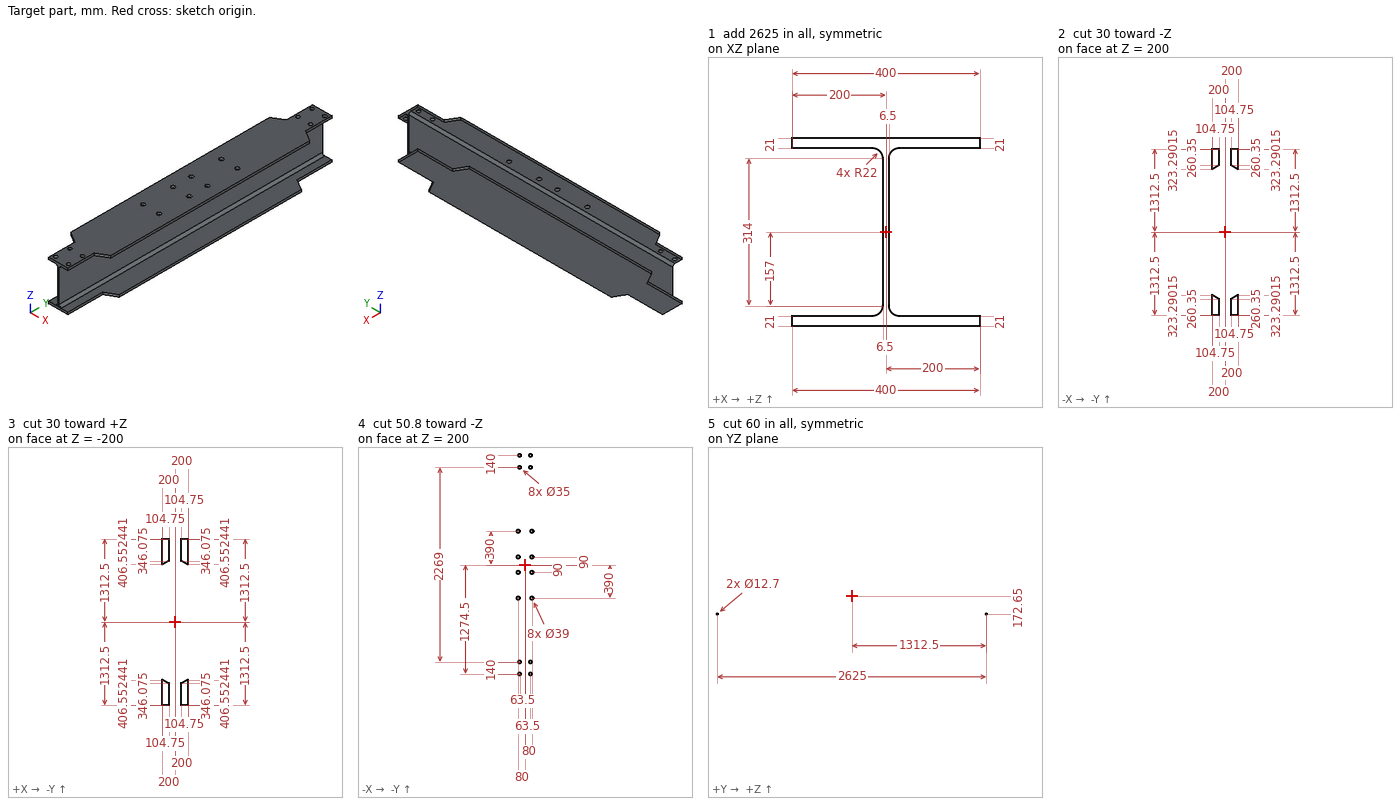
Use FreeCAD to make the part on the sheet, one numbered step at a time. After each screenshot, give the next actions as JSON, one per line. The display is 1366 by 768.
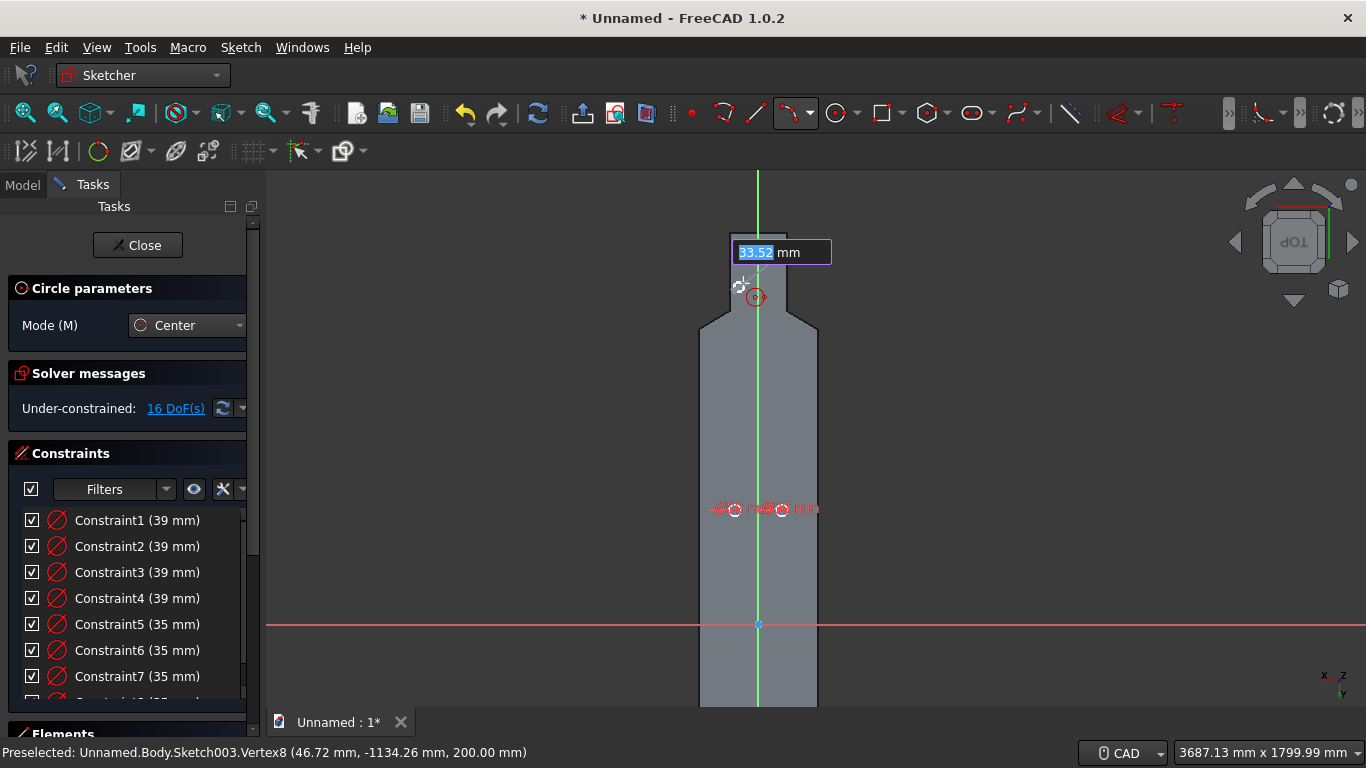
{"action": "type", "text": "35"}
{"action": "key", "text": "Return"}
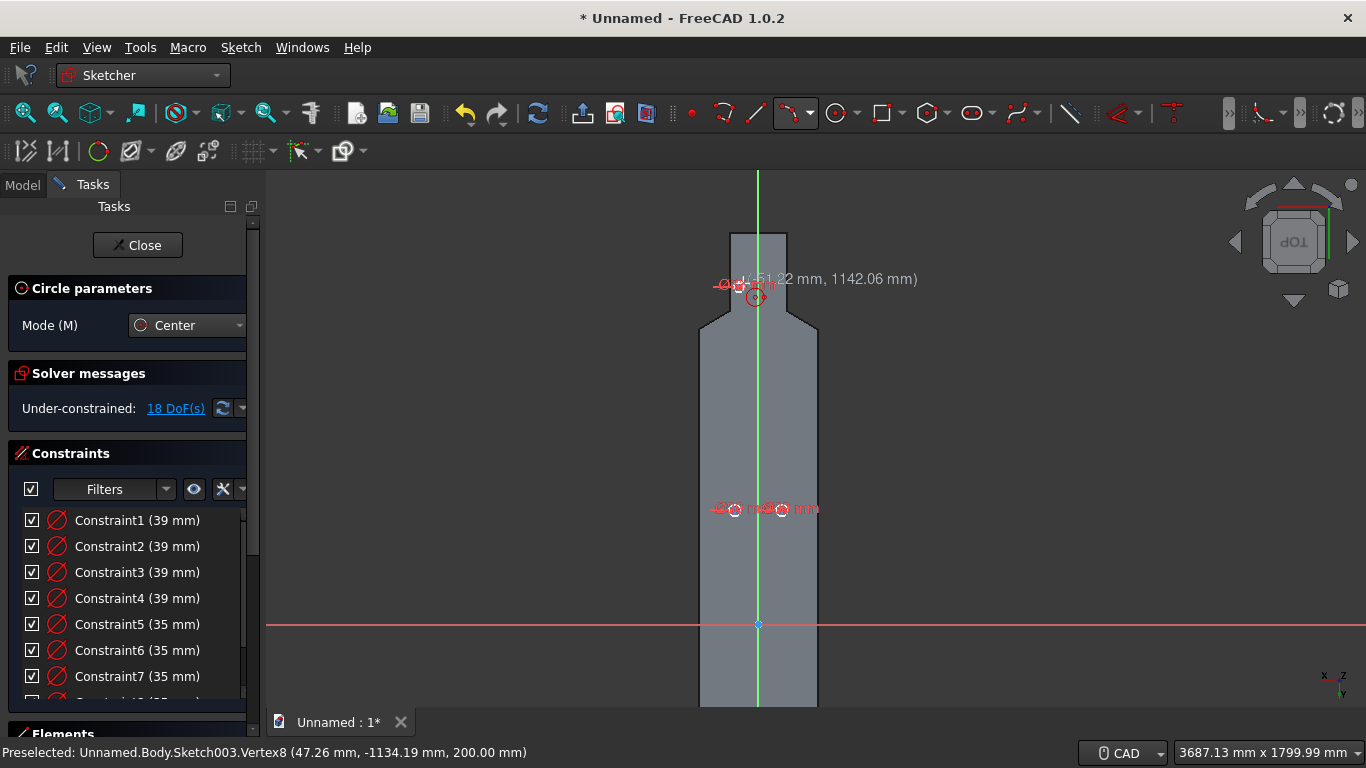
{"action": "scroll", "coordinate": [777, 286], "scroll_direction": "up", "scroll_amount": 8}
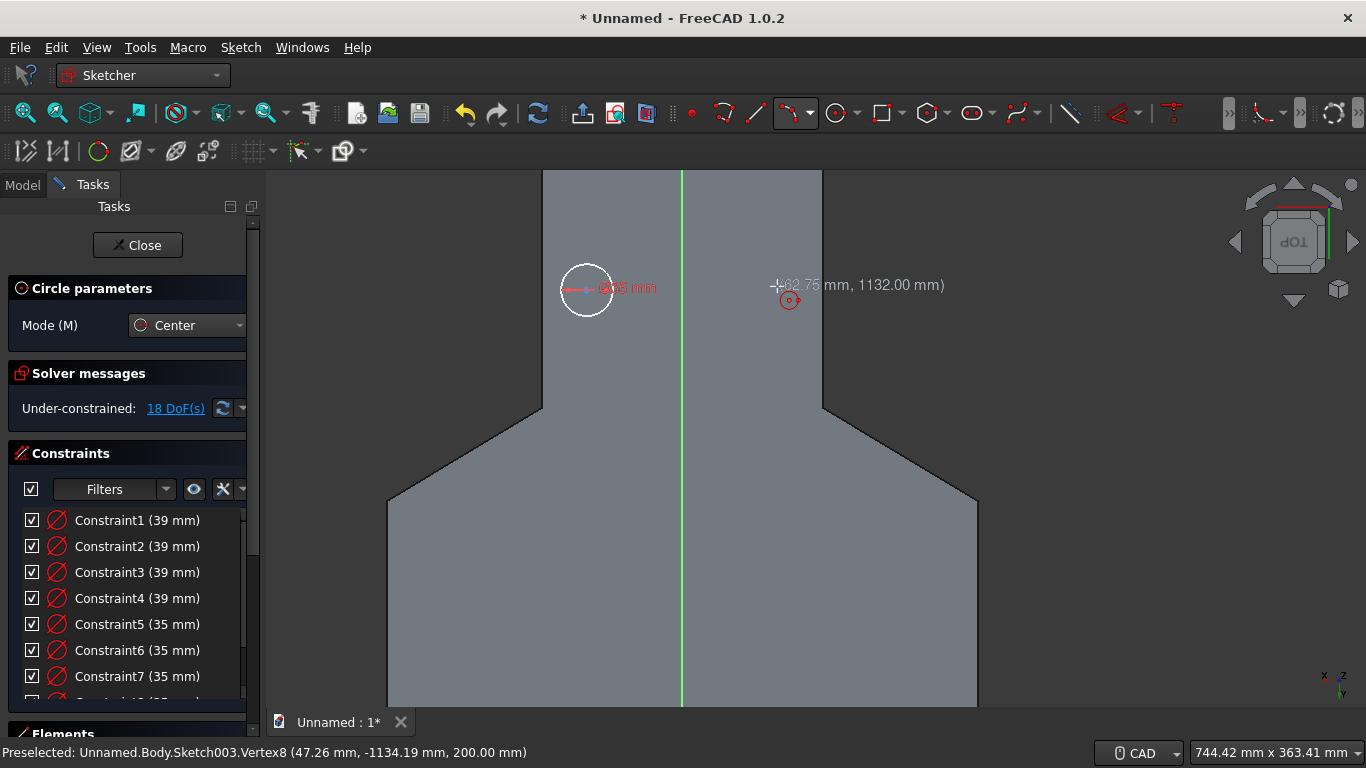
{"action": "scroll", "coordinate": [754, 286], "scroll_direction": "down", "scroll_amount": 12}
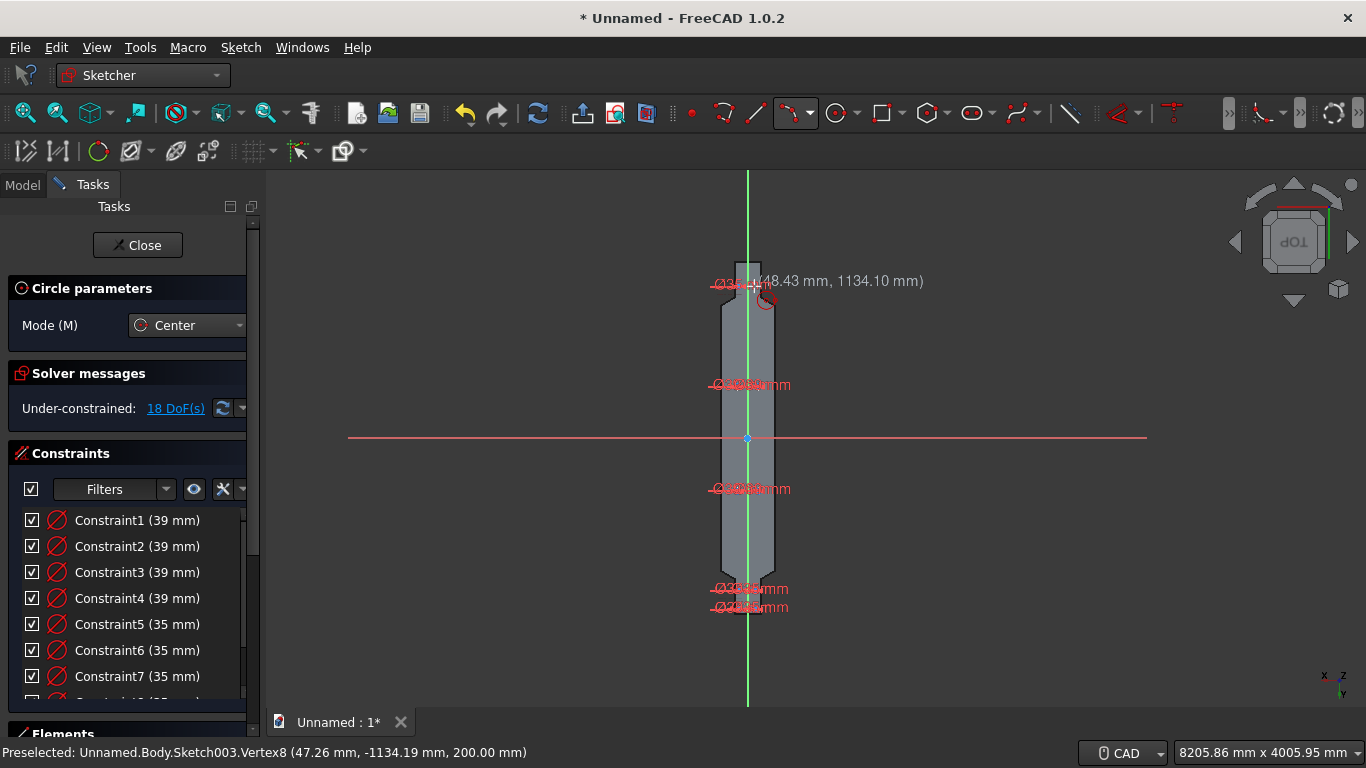
{"action": "scroll", "coordinate": [756, 286], "scroll_direction": "up", "scroll_amount": 4}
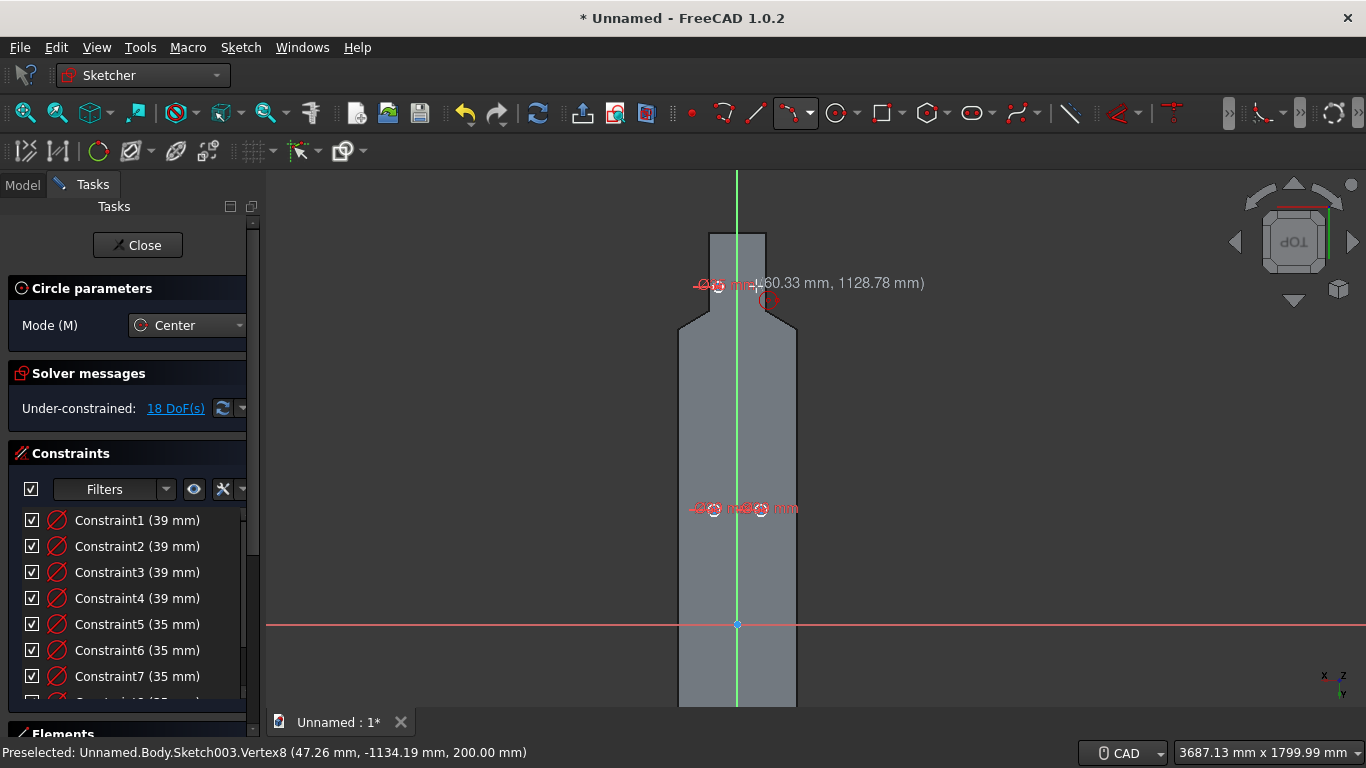
{"action": "left_click", "coordinate": [756, 286]}
{"action": "mouse_move", "coordinate": [760, 283]}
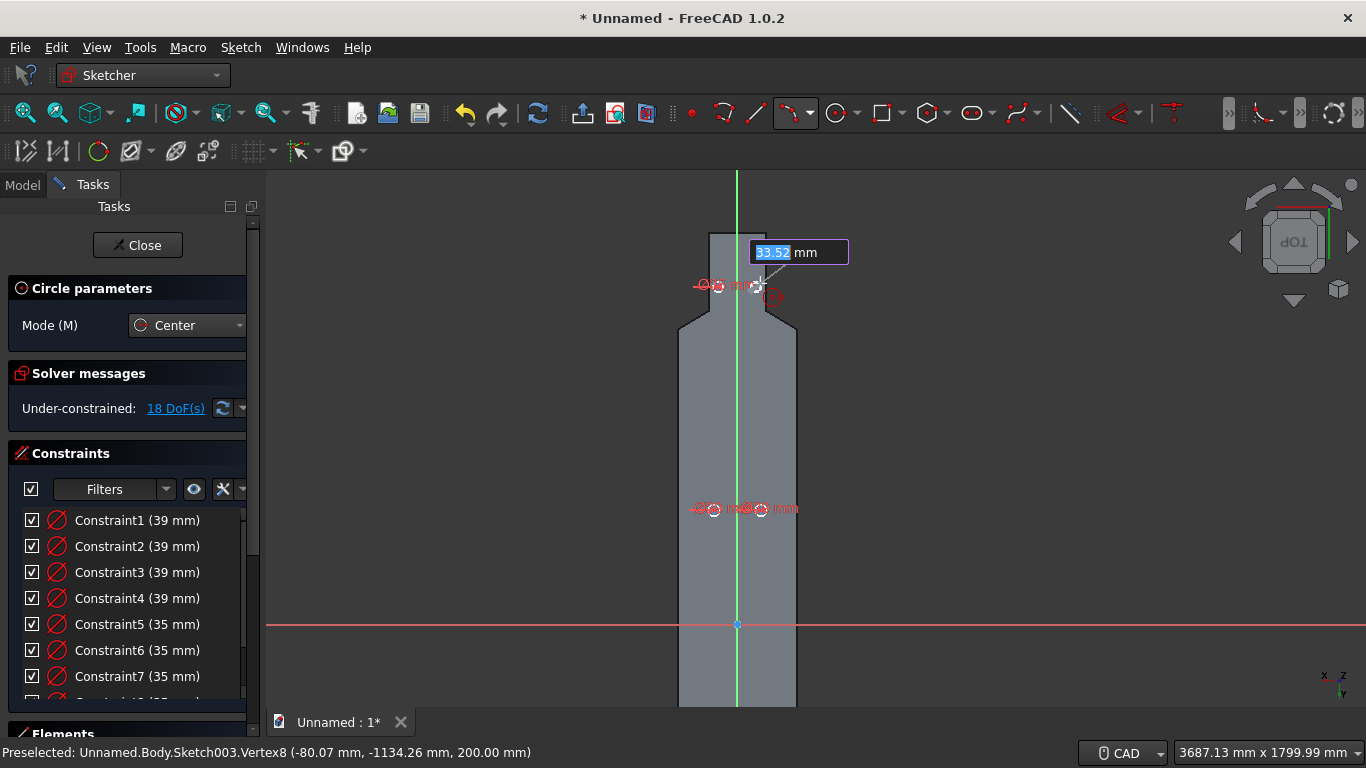
{"action": "type", "text": "35"}
{"action": "key", "text": "Return"}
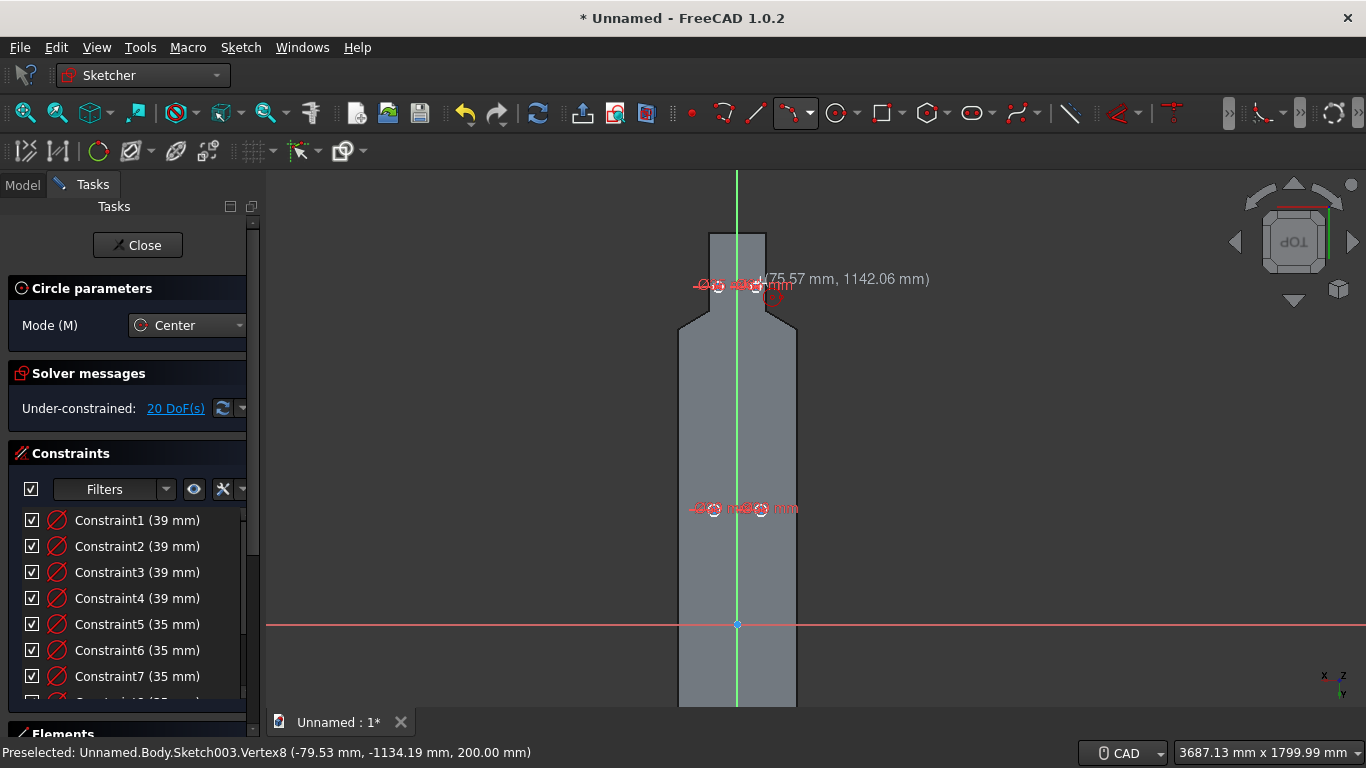
{"action": "scroll", "coordinate": [719, 244], "scroll_direction": "up", "scroll_amount": 8}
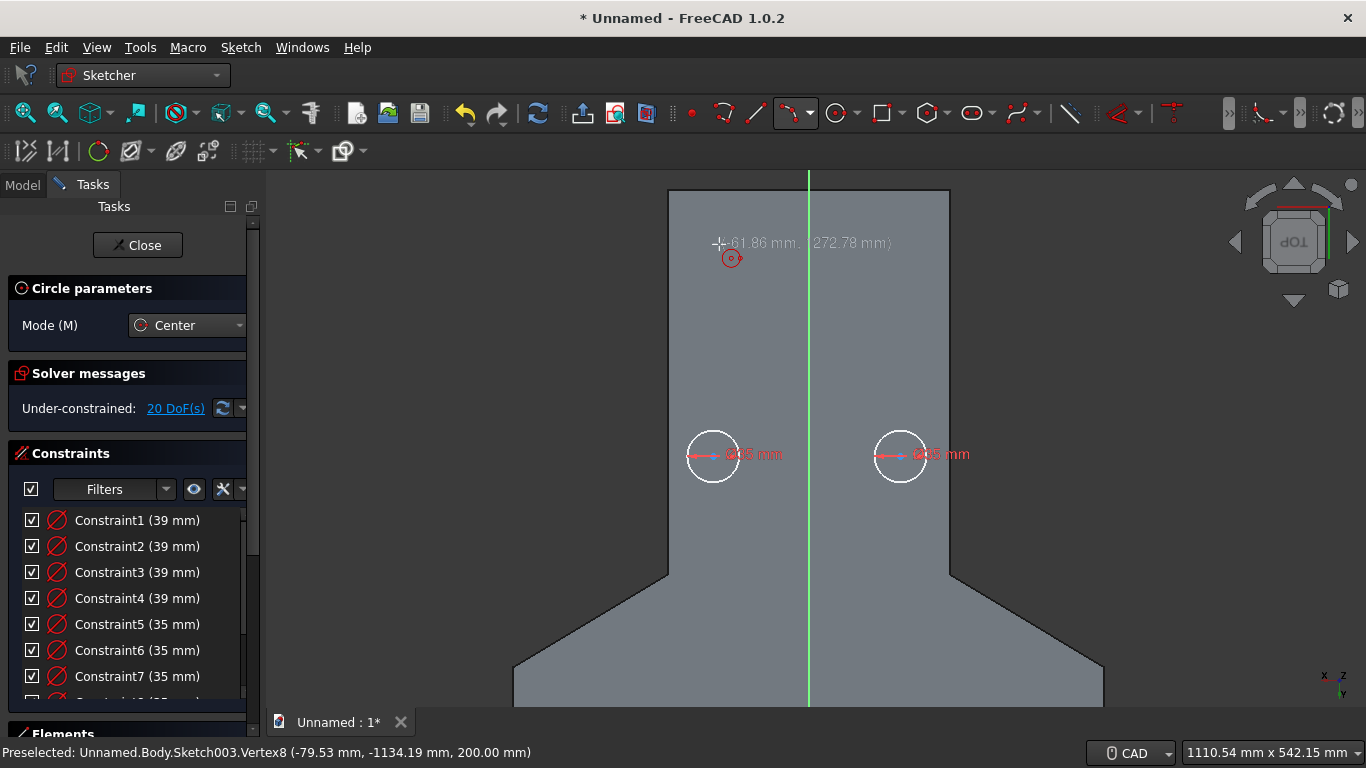
{"action": "scroll", "coordinate": [741, 270], "scroll_direction": "down", "scroll_amount": 12}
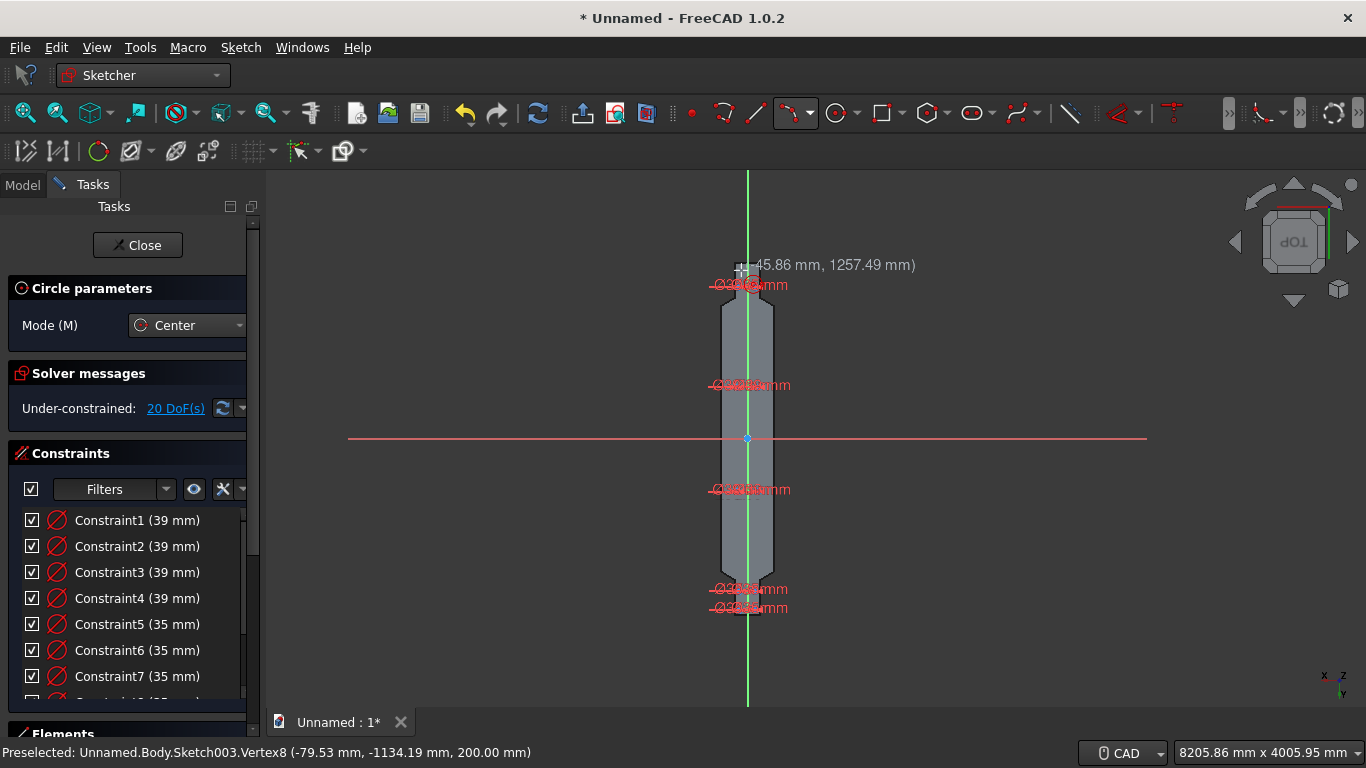
{"action": "scroll", "coordinate": [739, 268], "scroll_direction": "up", "scroll_amount": 4}